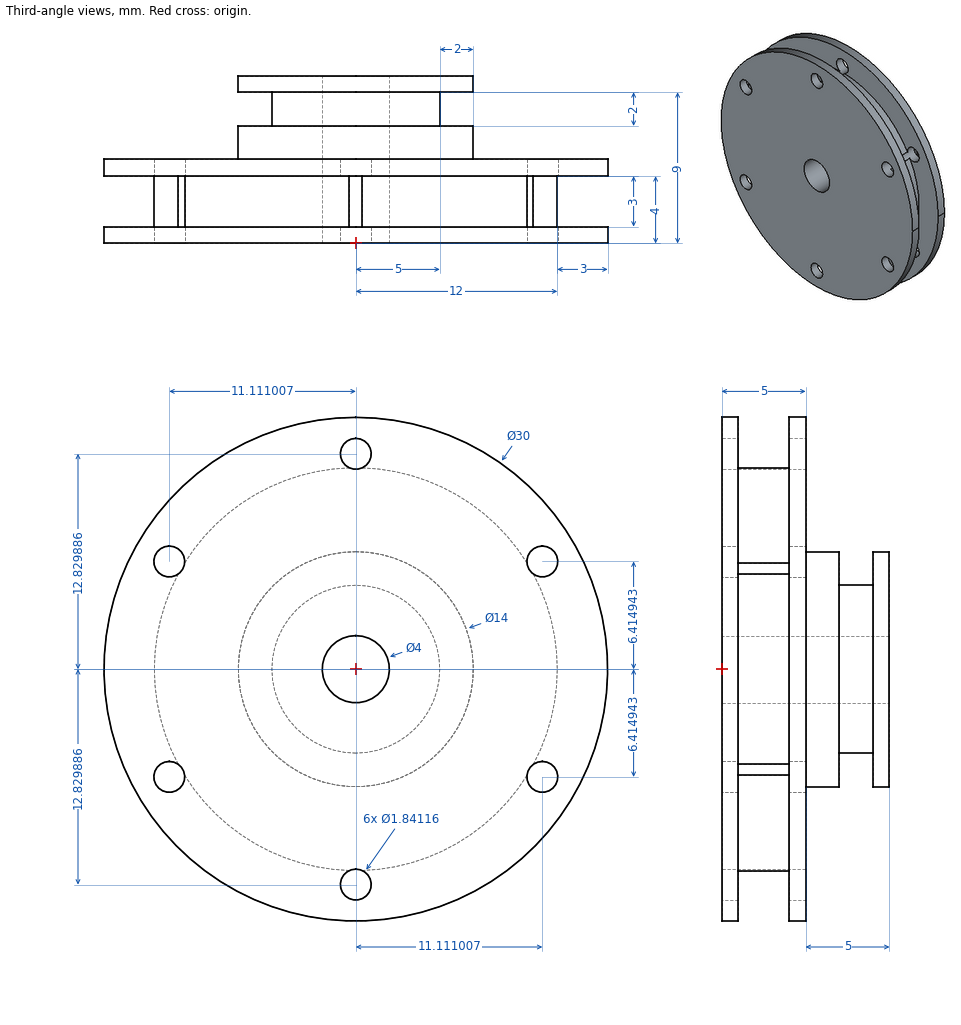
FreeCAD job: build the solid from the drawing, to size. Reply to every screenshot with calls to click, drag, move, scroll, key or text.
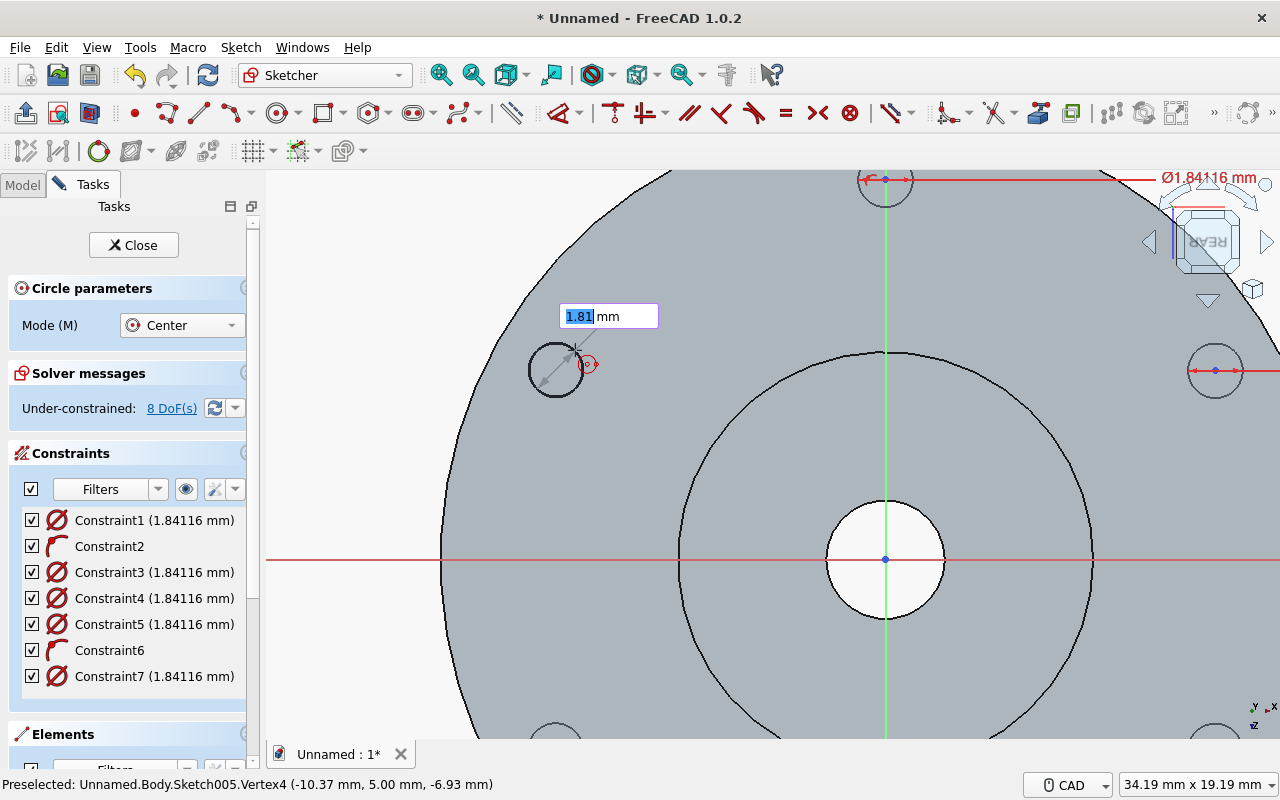
text(1.84116)
key(Return)
key(Escape)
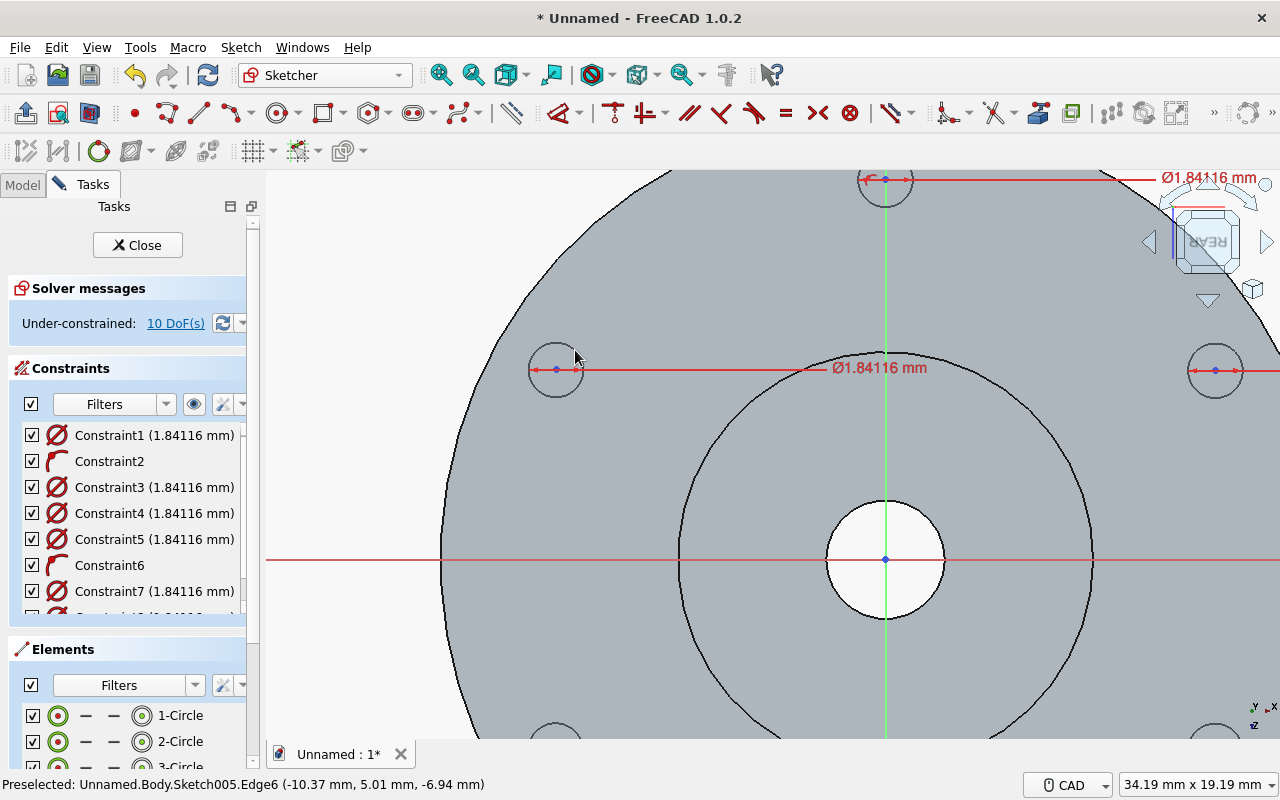
scroll(557, 369, down, 4)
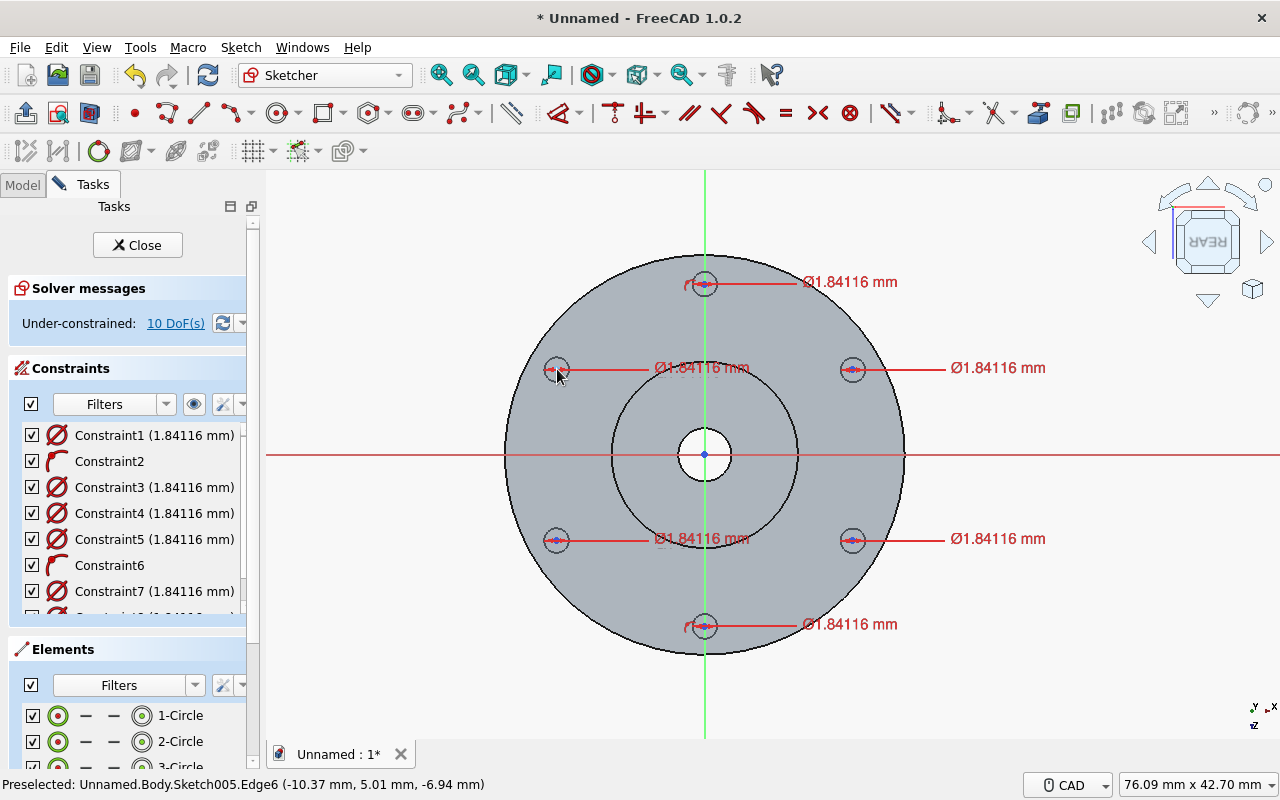
click(853, 370)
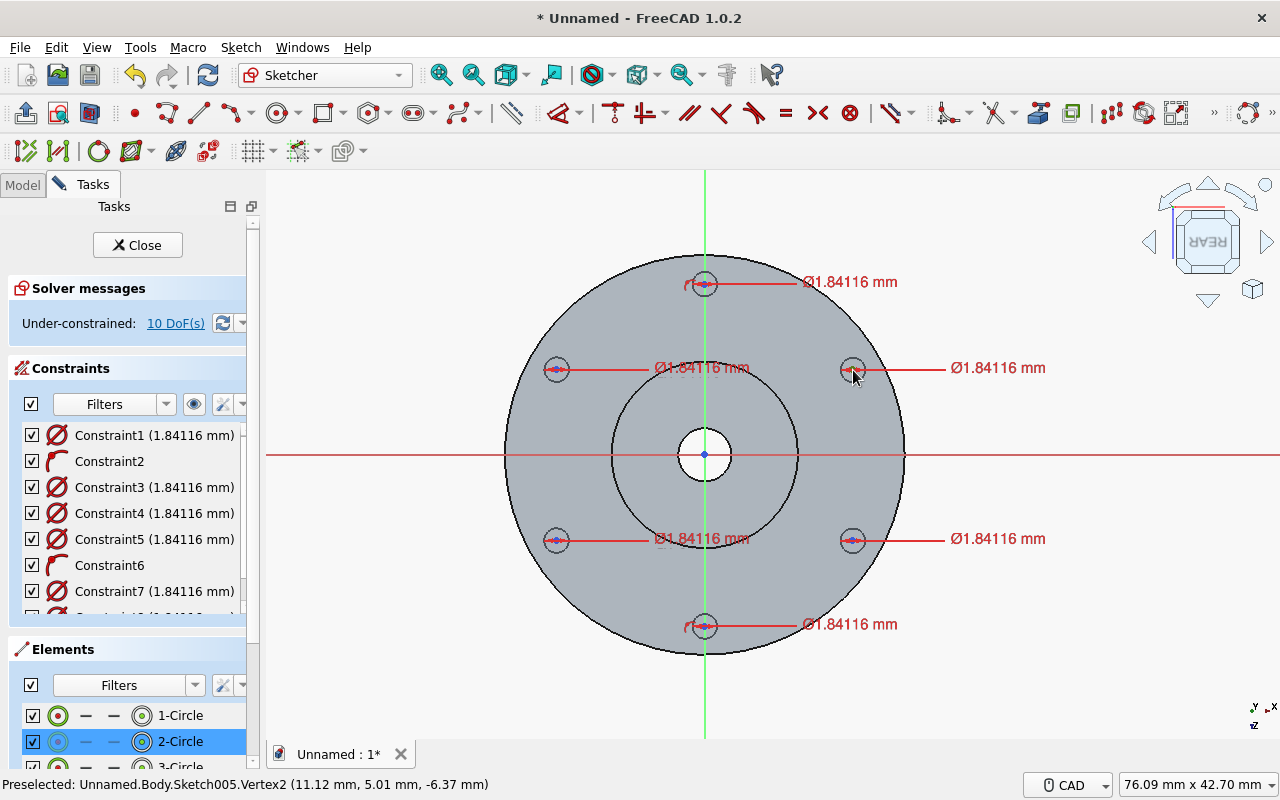
click(853, 541)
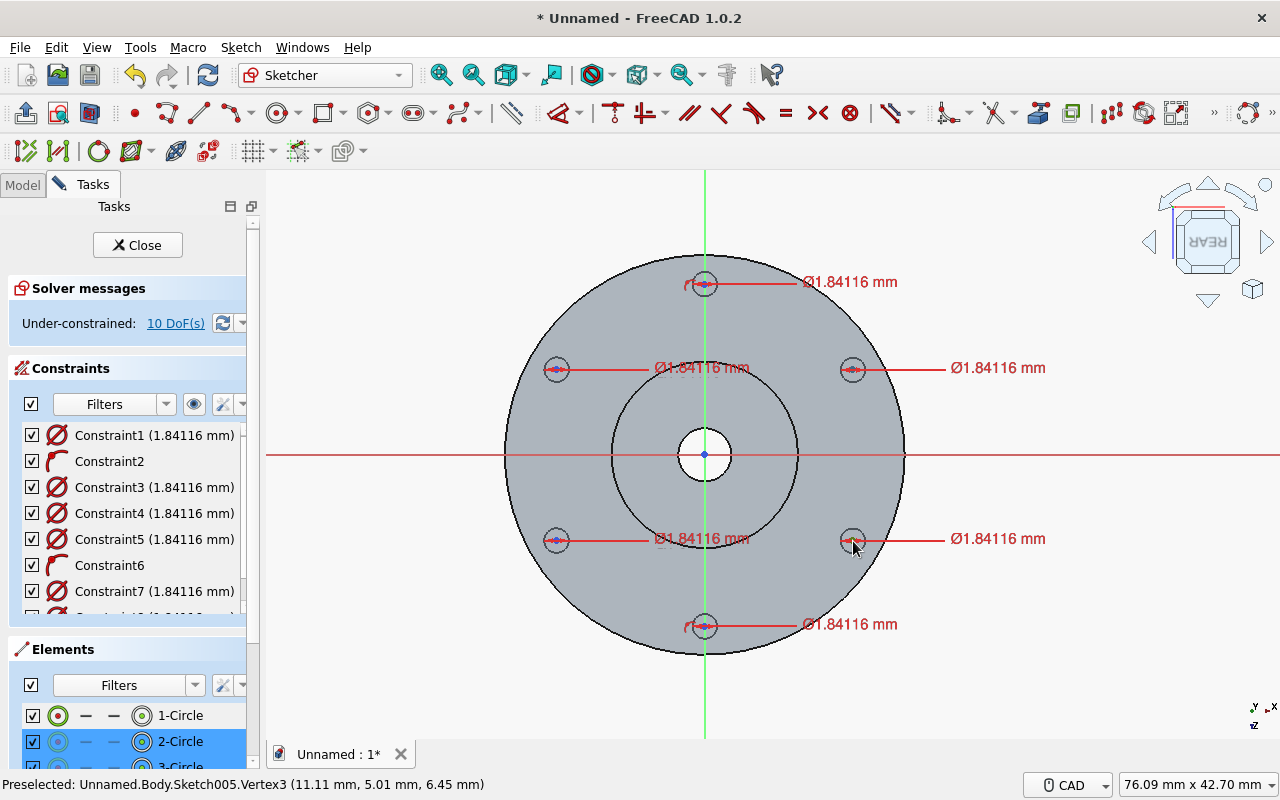
key(v)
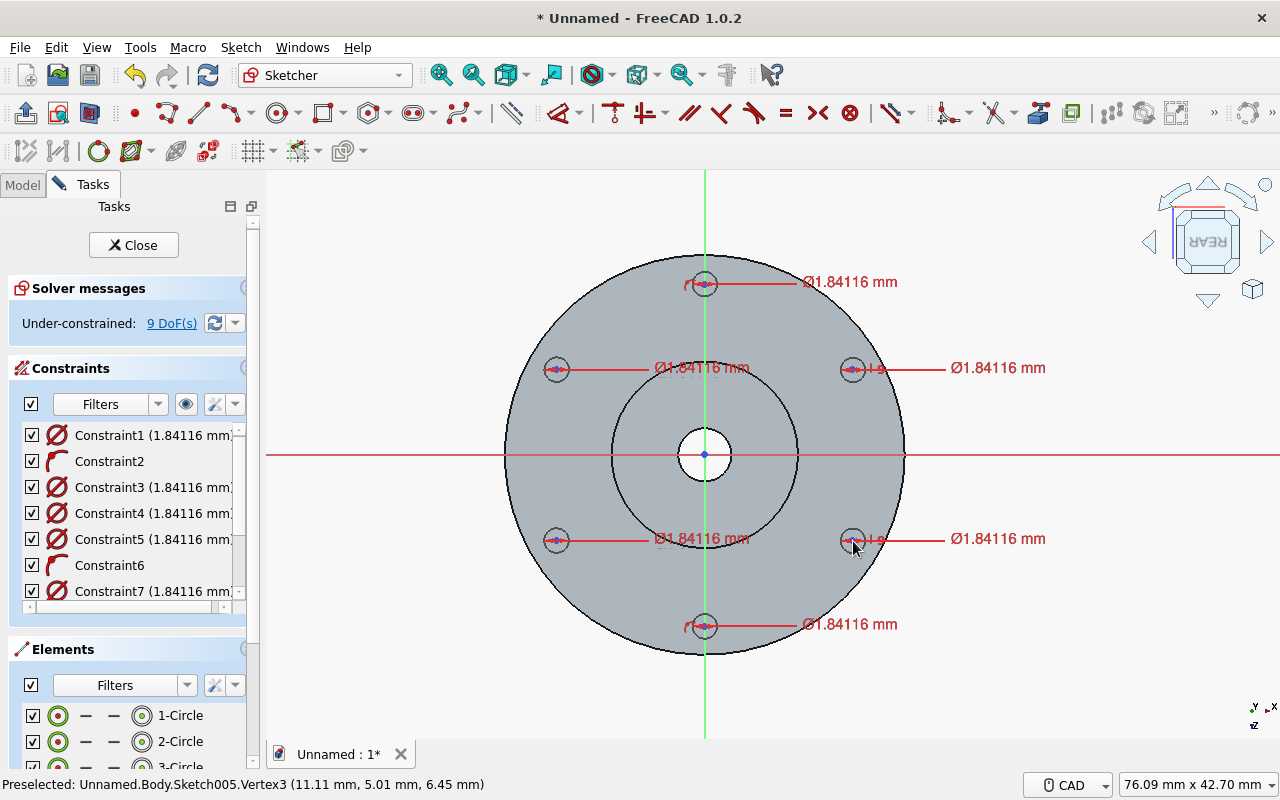
click(853, 541)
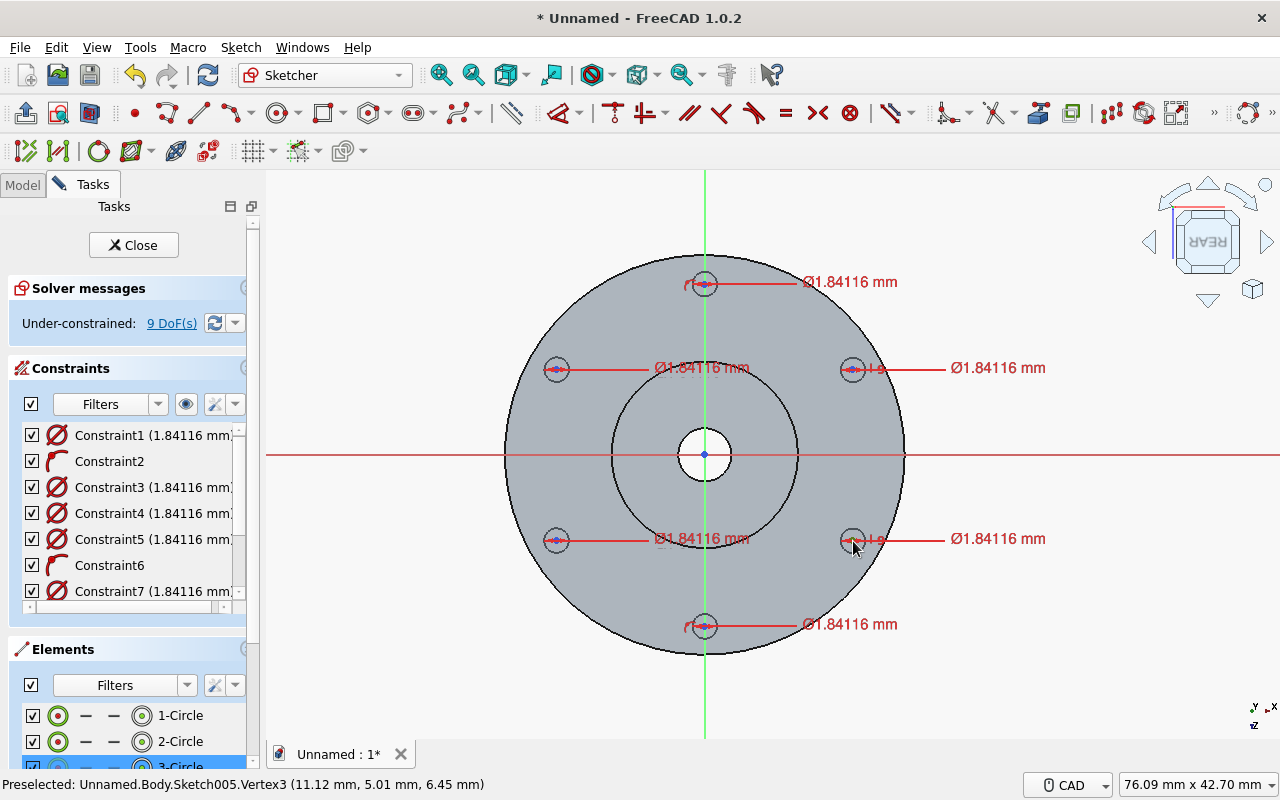
click(557, 541)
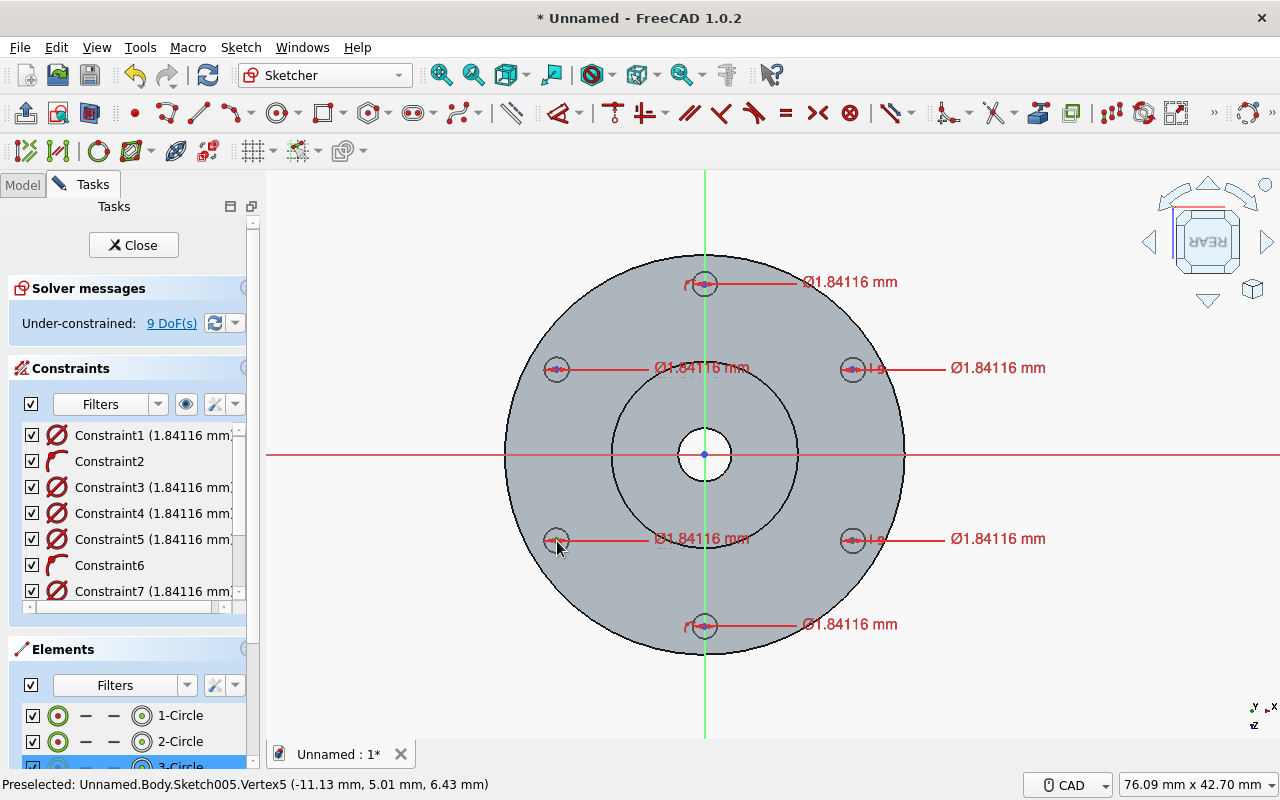
click(668, 114)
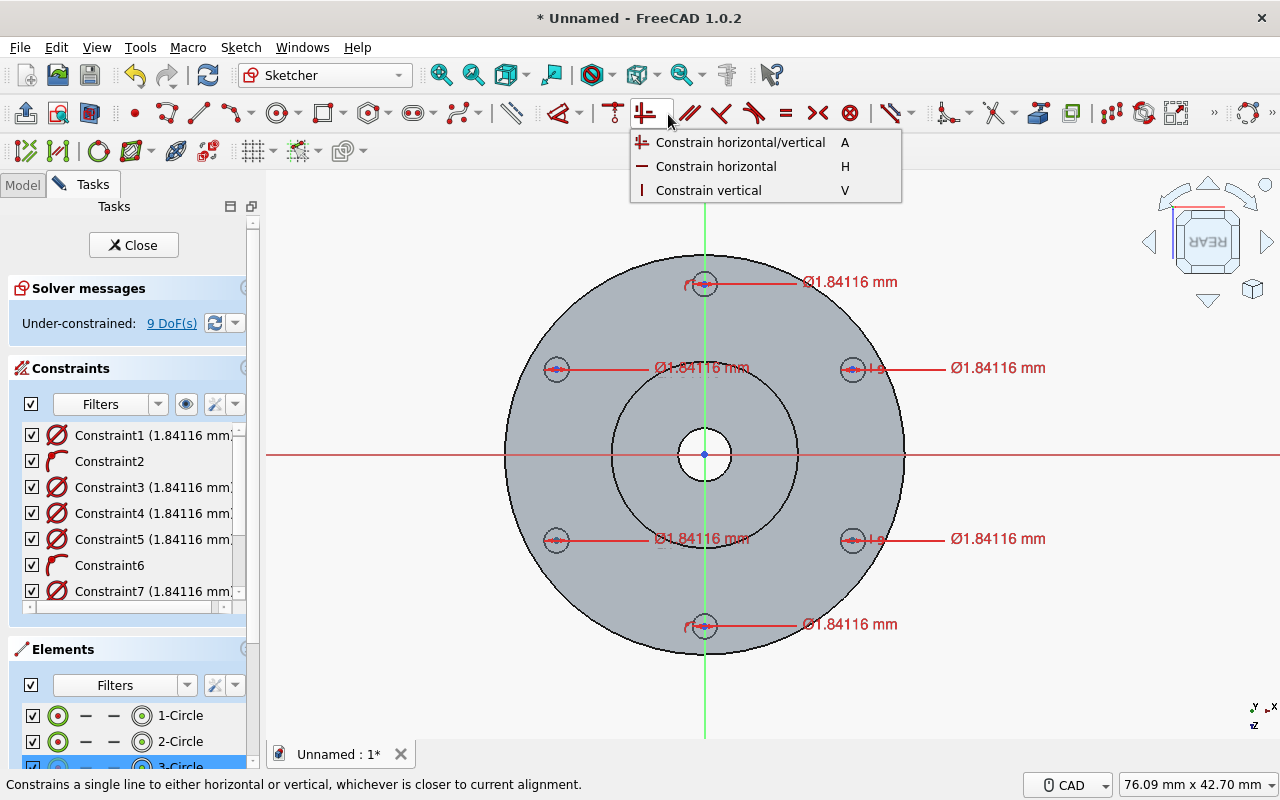
click(766, 166)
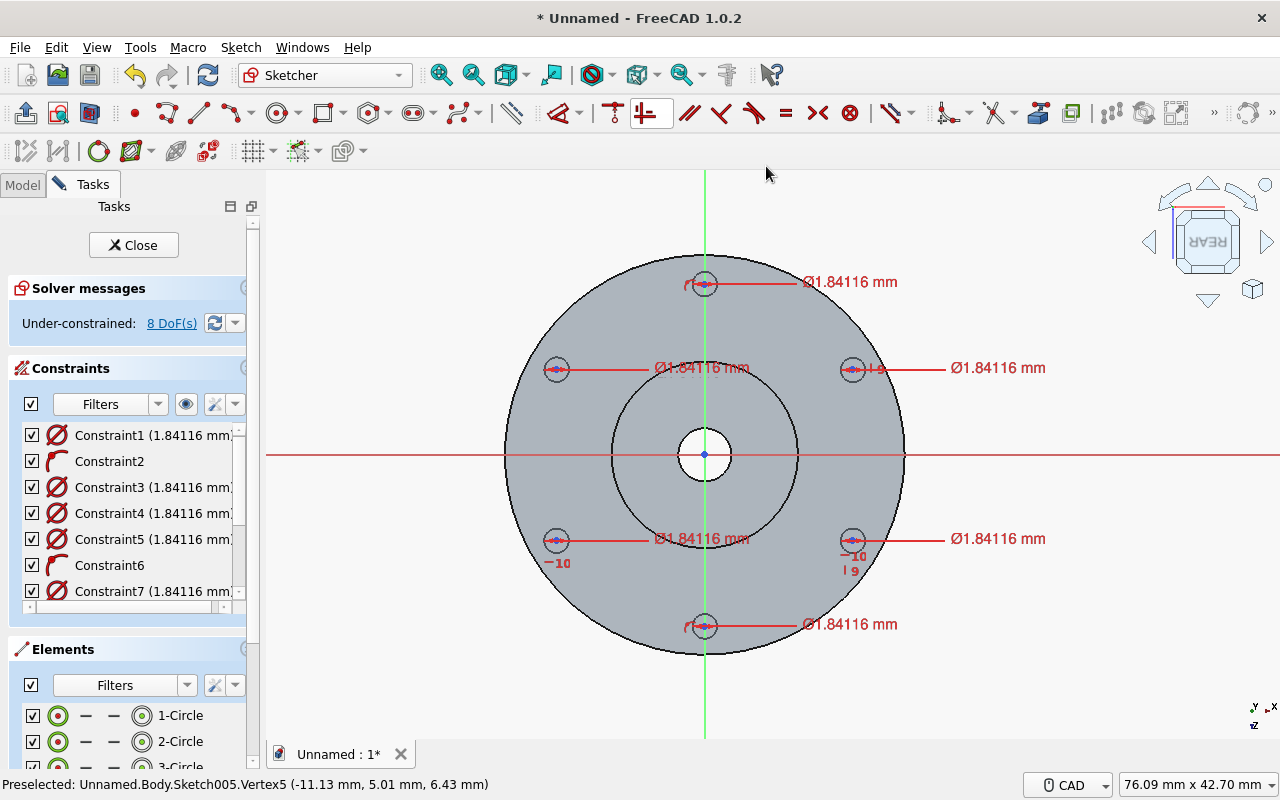
click(557, 541)